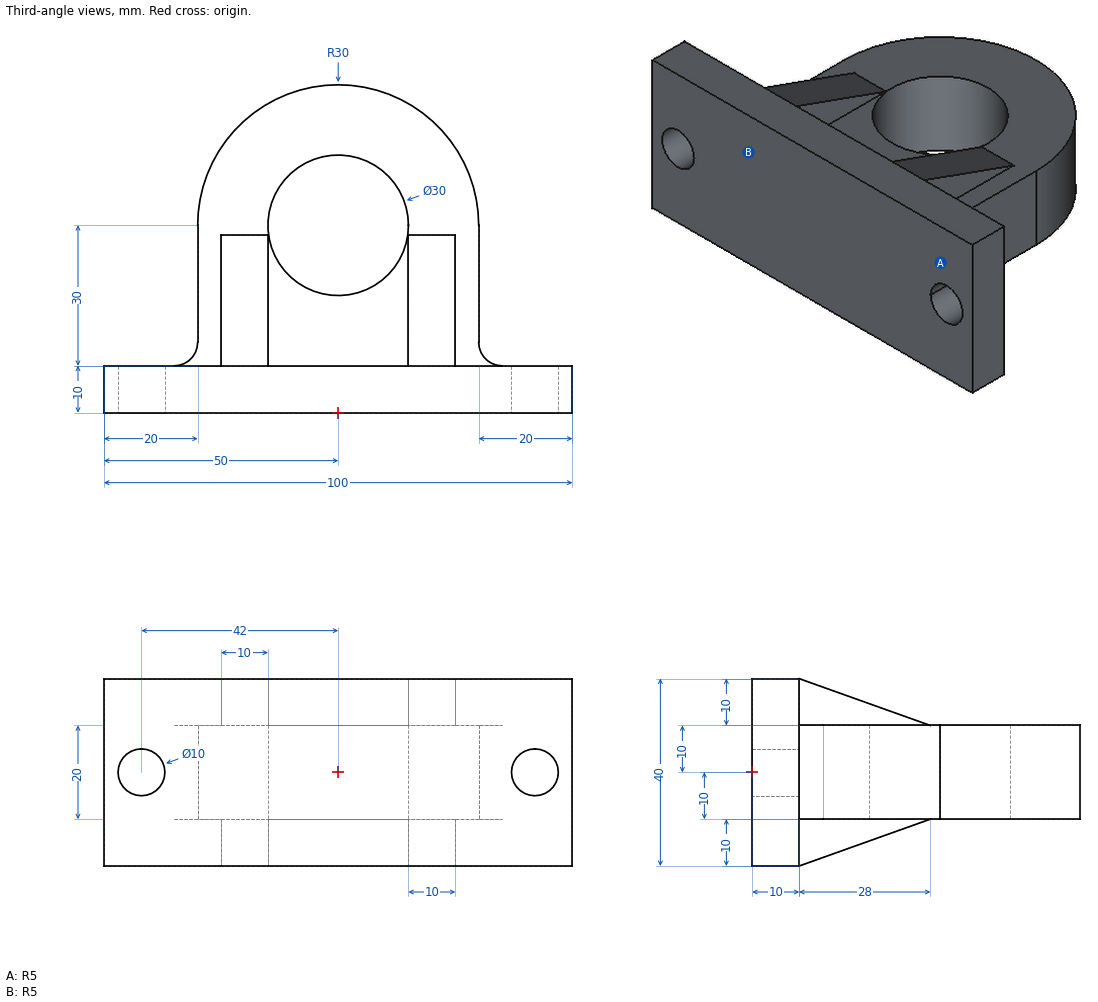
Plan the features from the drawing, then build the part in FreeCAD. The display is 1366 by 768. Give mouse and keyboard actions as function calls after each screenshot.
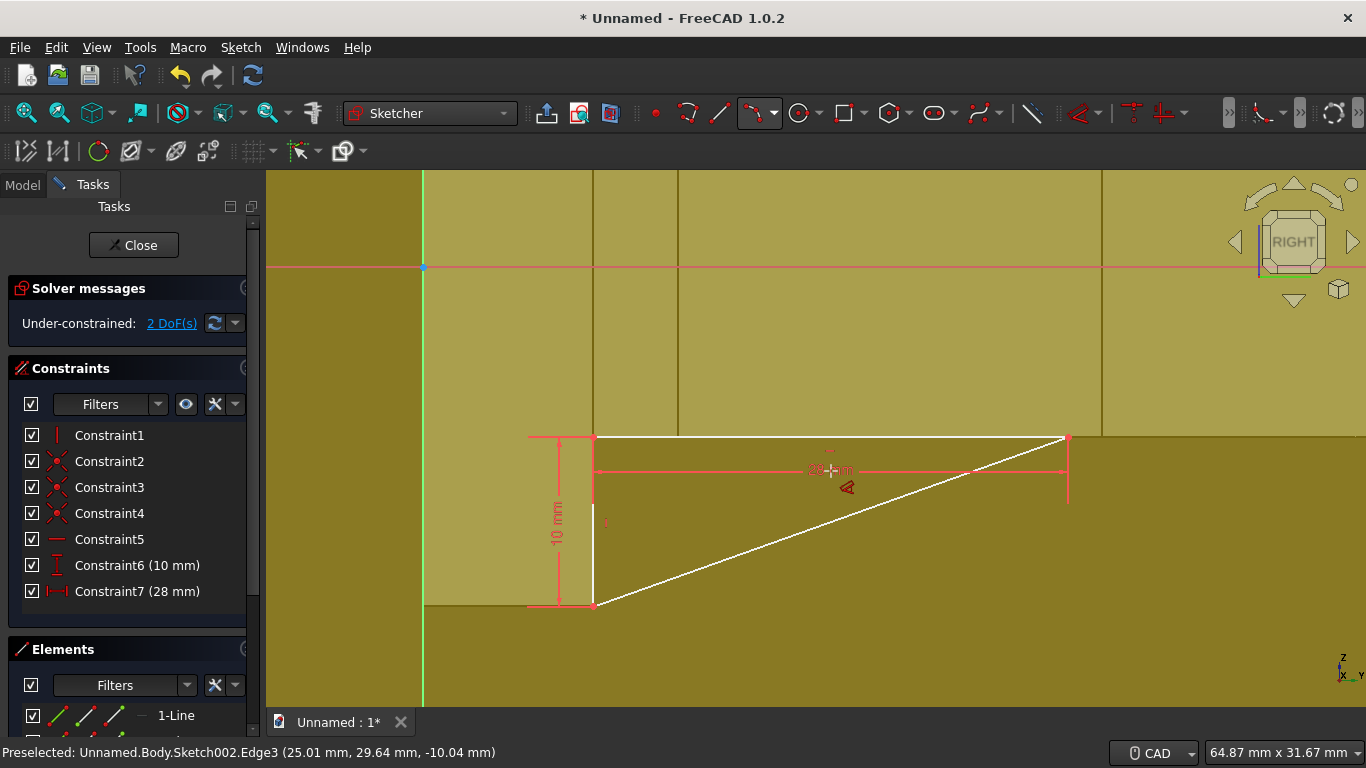
click(593, 437)
click(508, 233)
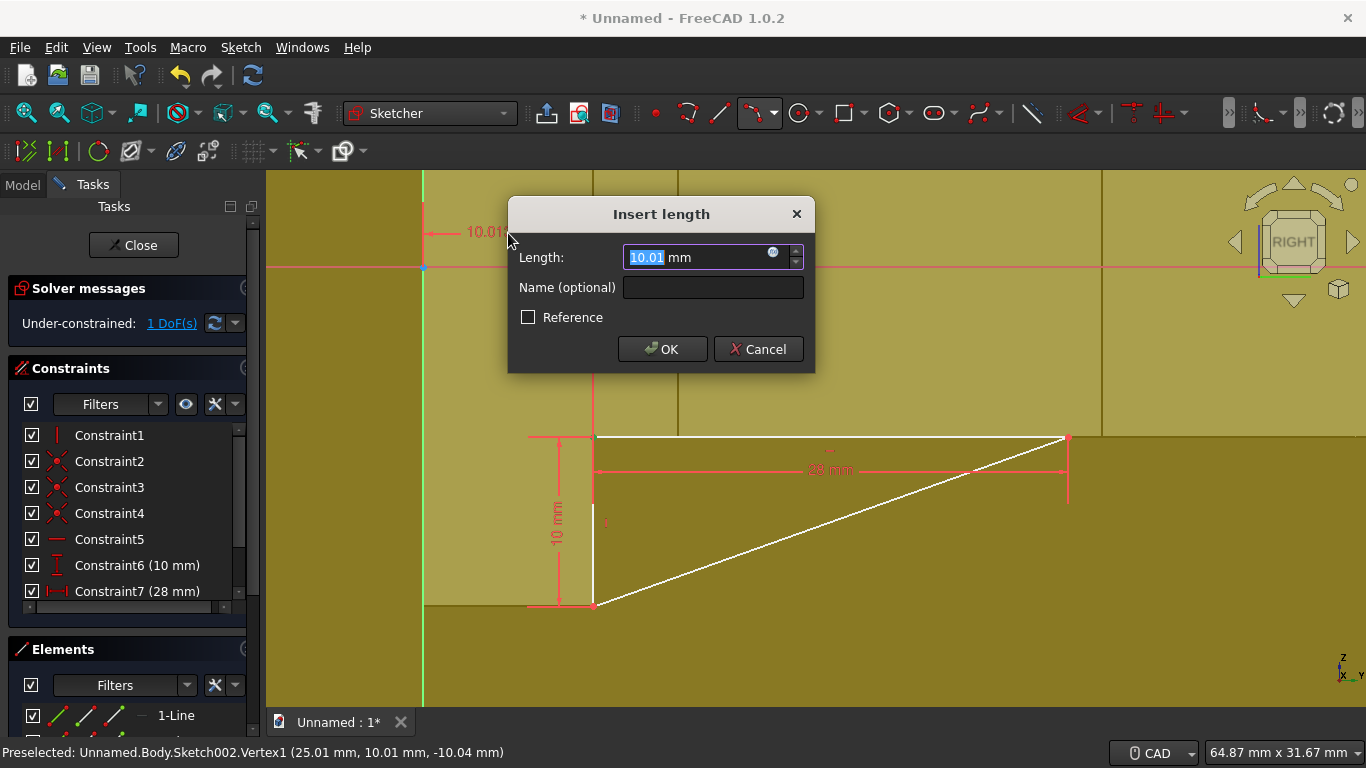
text(10)
key(Return)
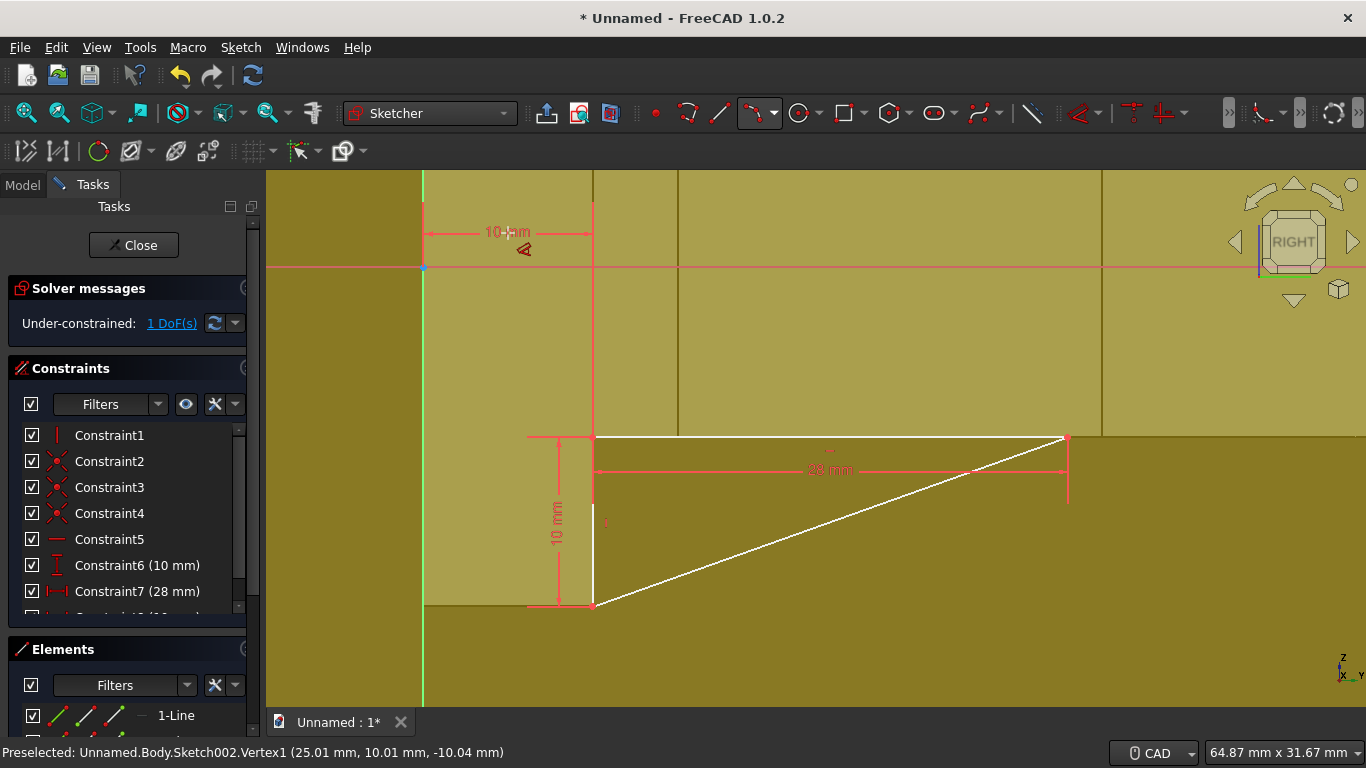
click(593, 437)
click(389, 352)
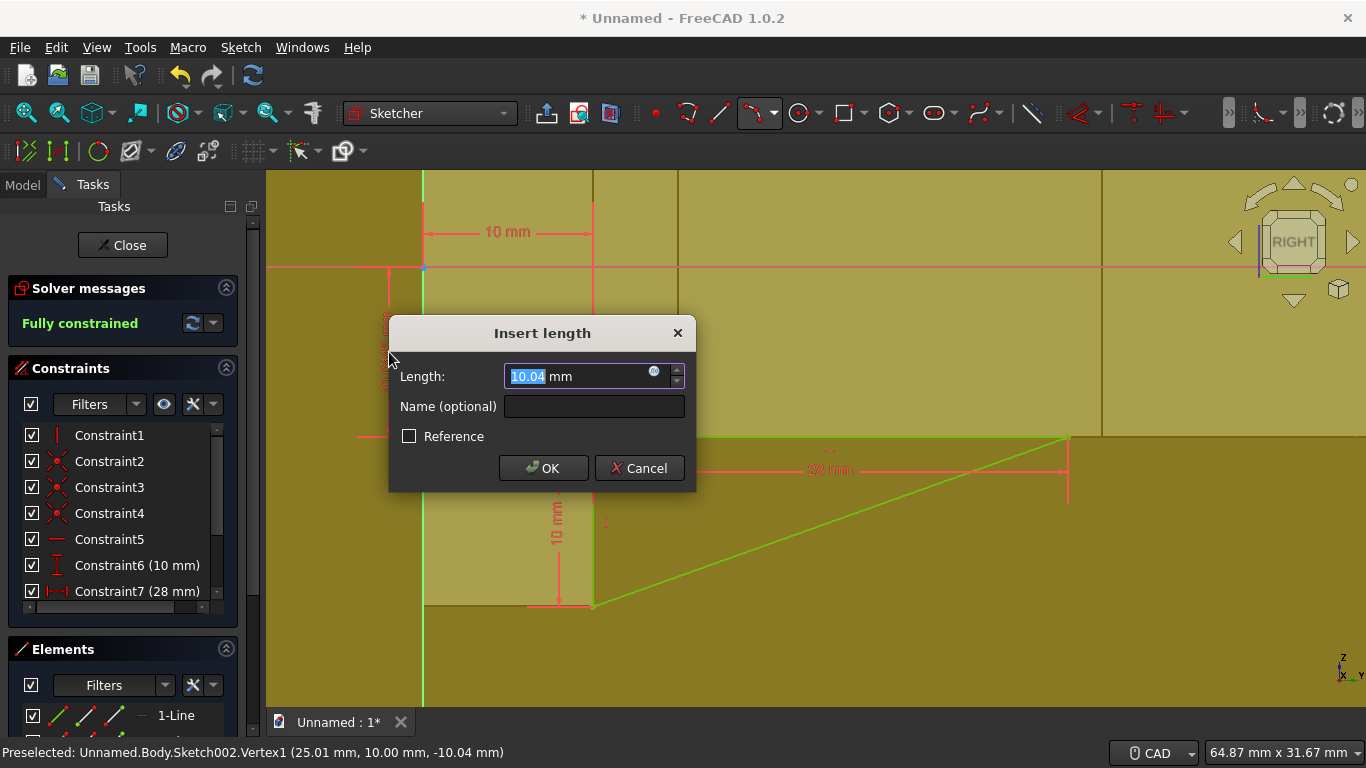
text(10)
key(Return)
key(Escape)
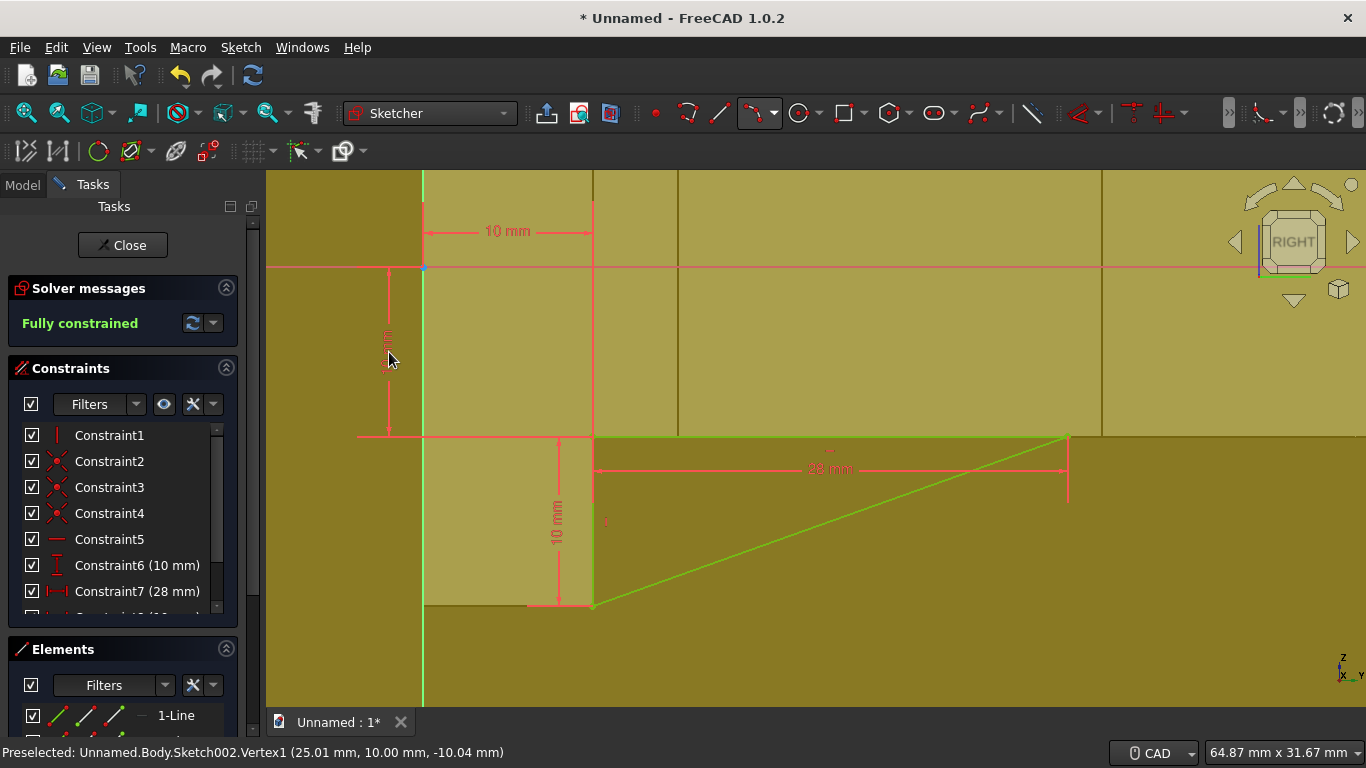
click(123, 245)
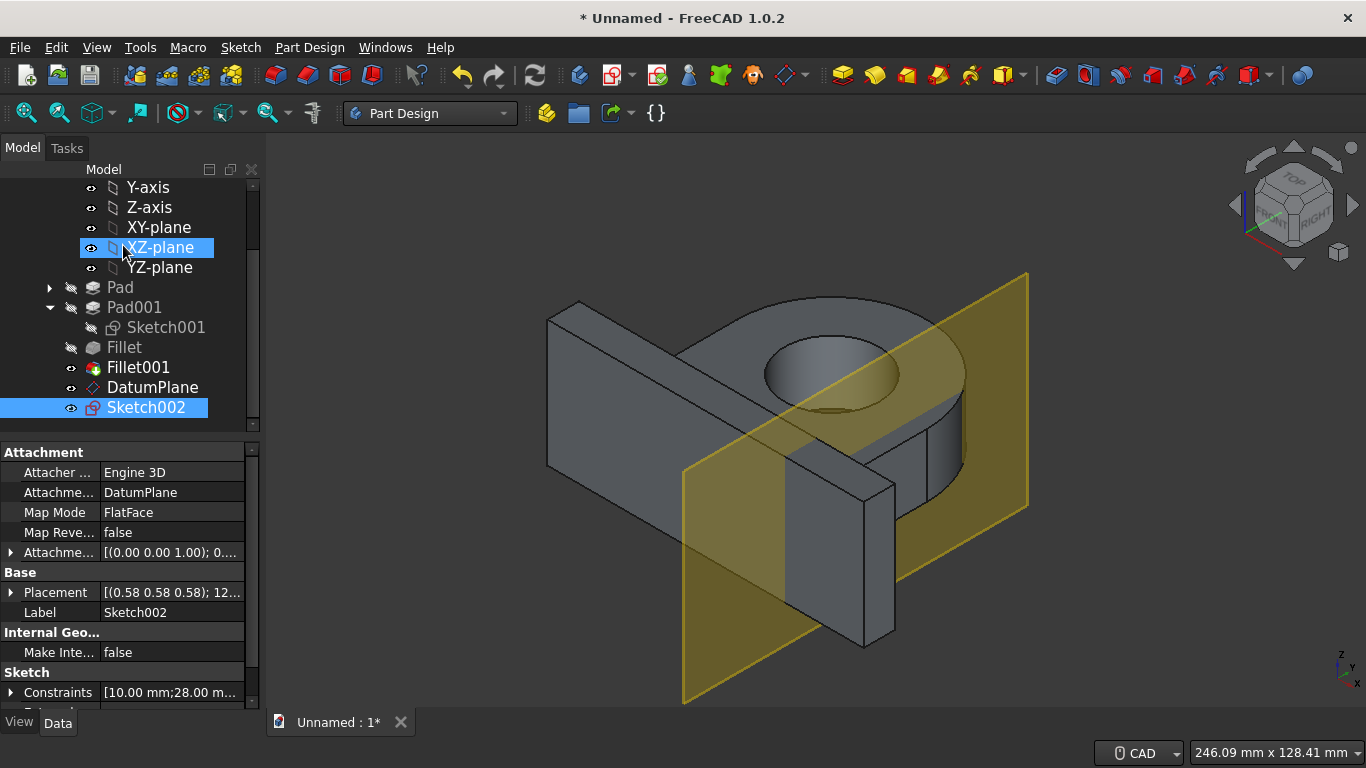
click(844, 76)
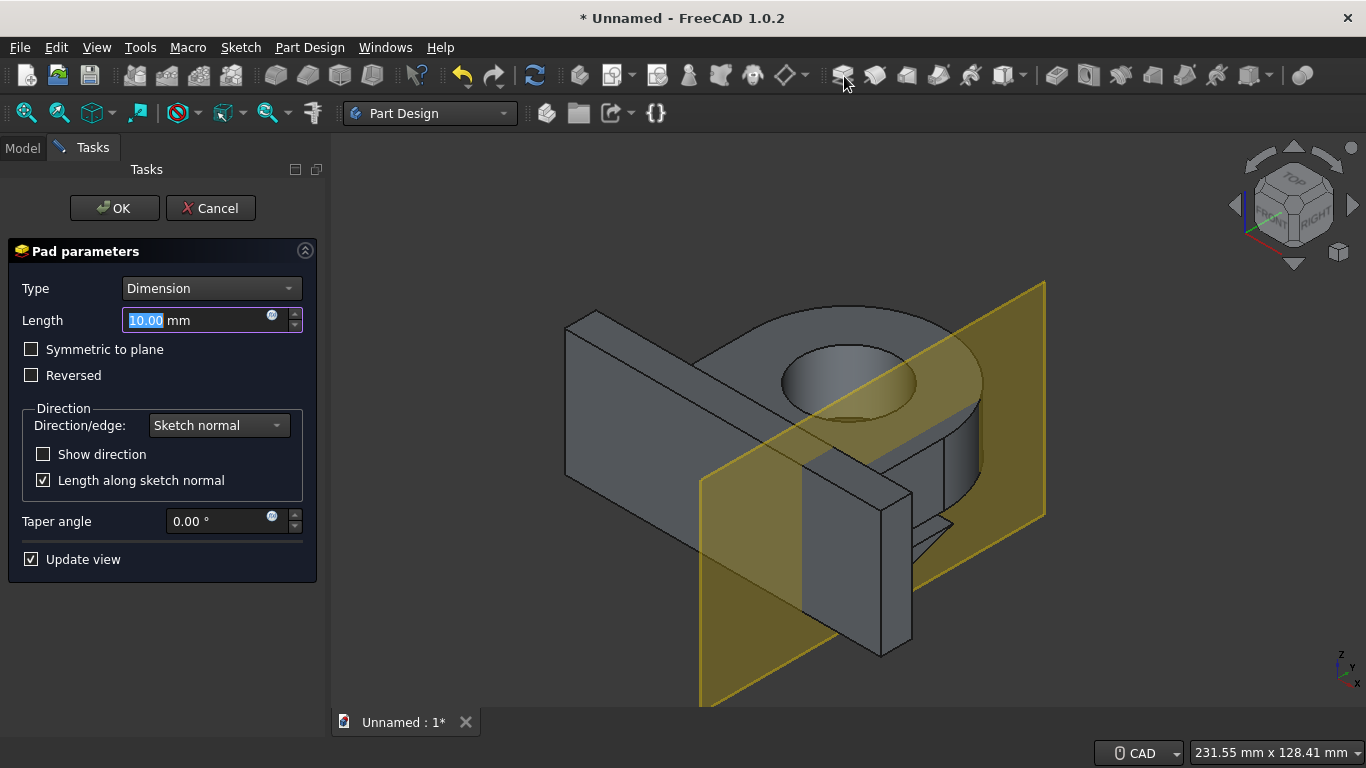
text(10)
key(Tab)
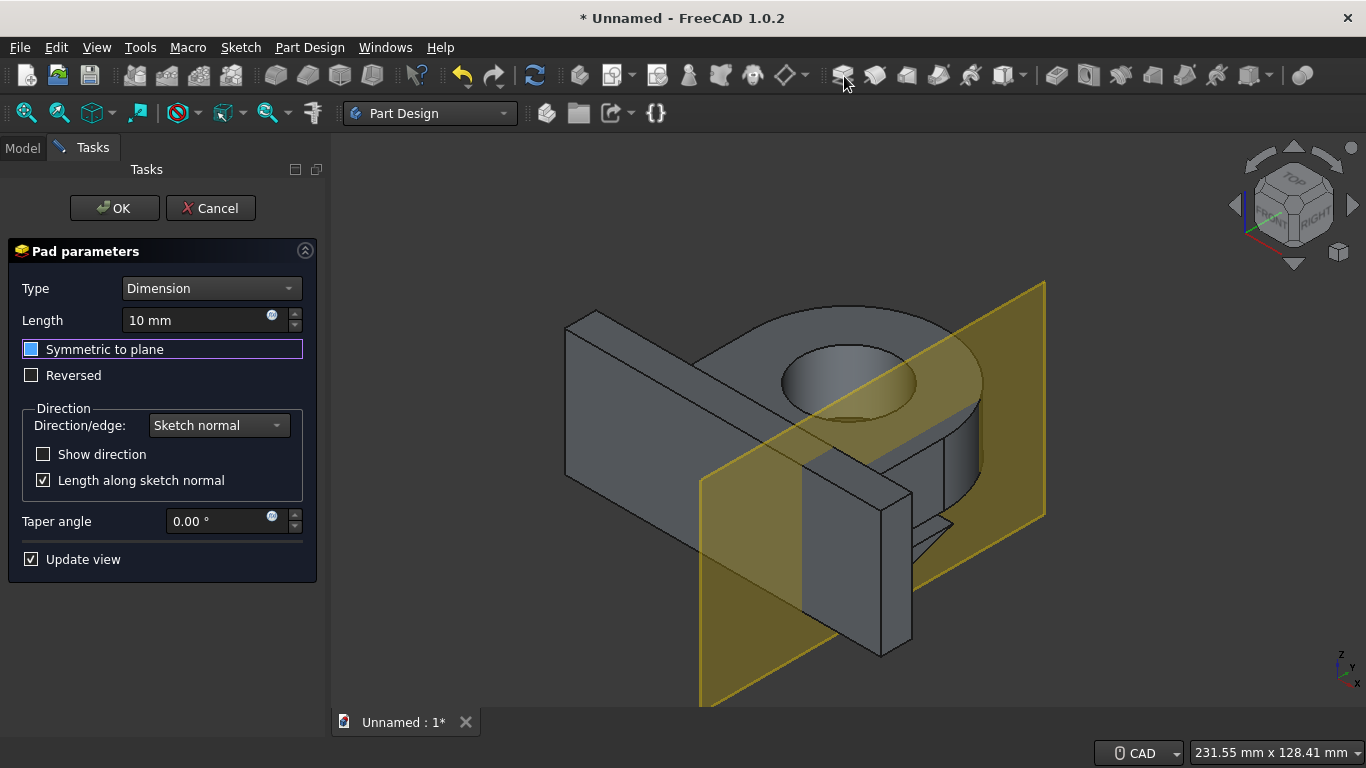
click(30, 375)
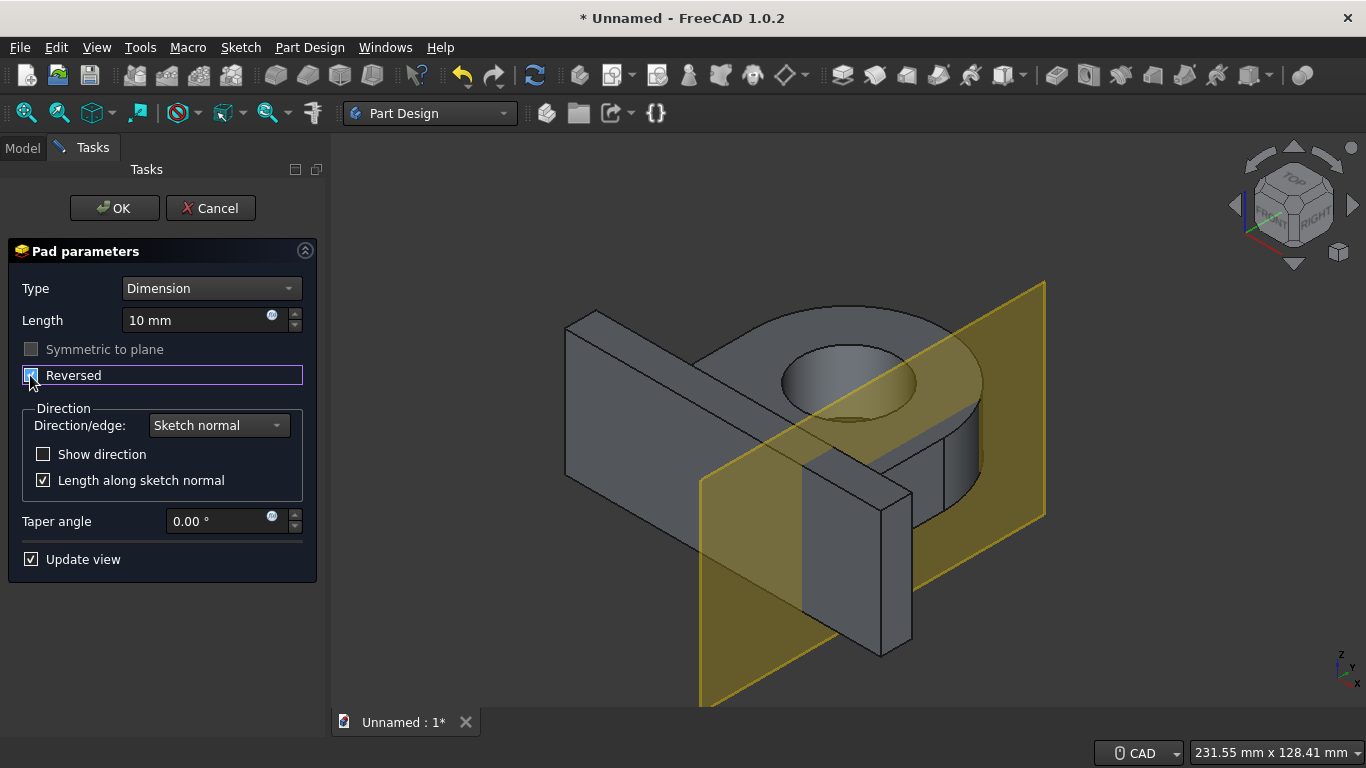
click(115, 208)